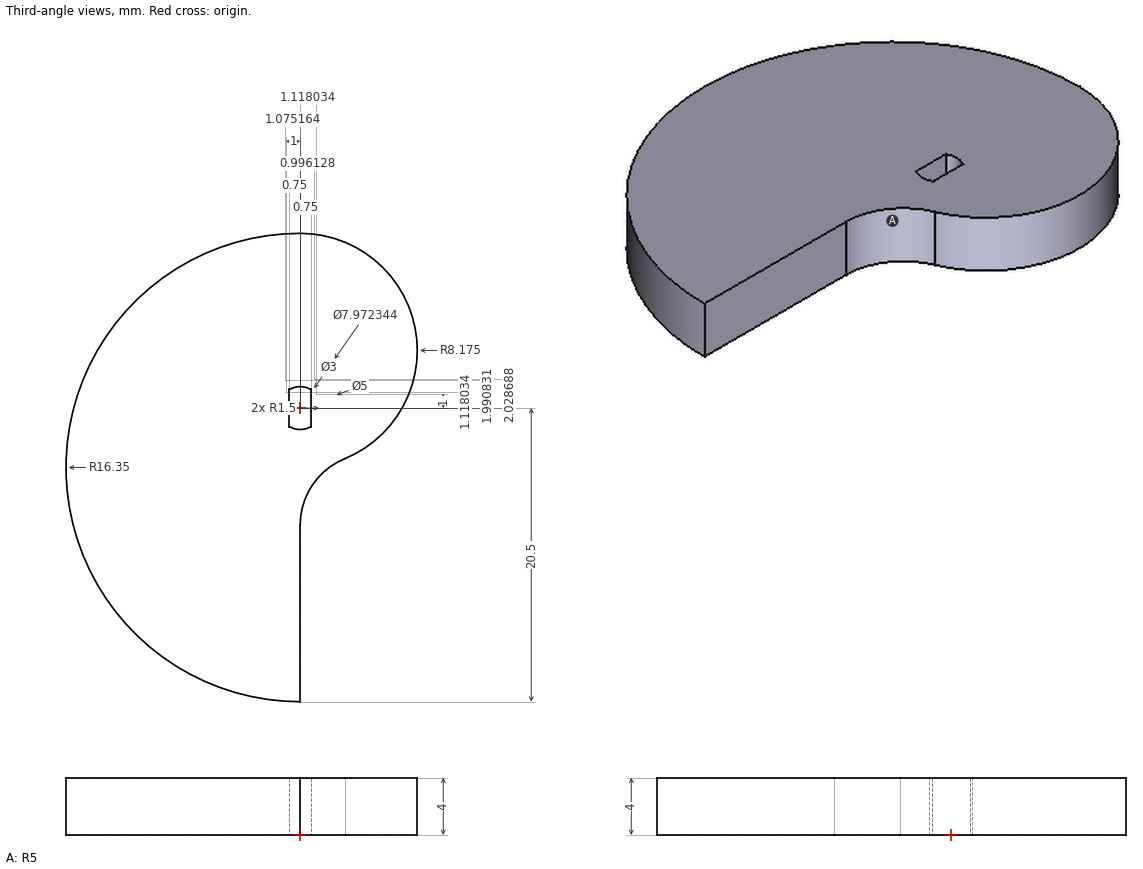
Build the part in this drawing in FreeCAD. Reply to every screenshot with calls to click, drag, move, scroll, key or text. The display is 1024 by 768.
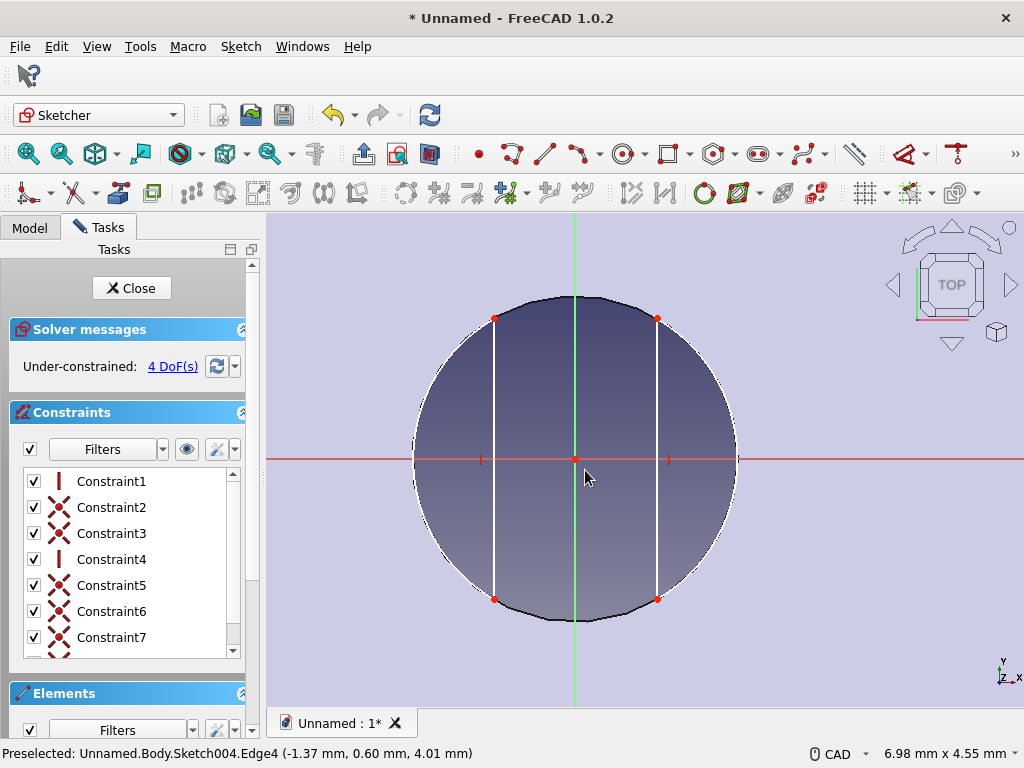
click(724, 525)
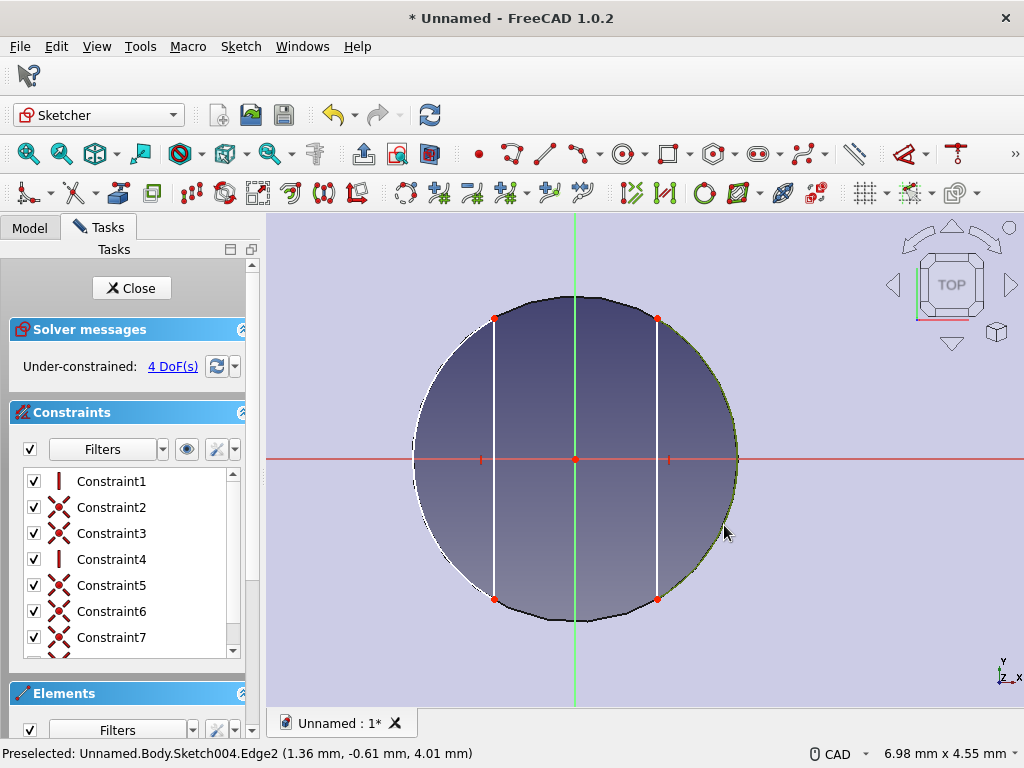
click(427, 393)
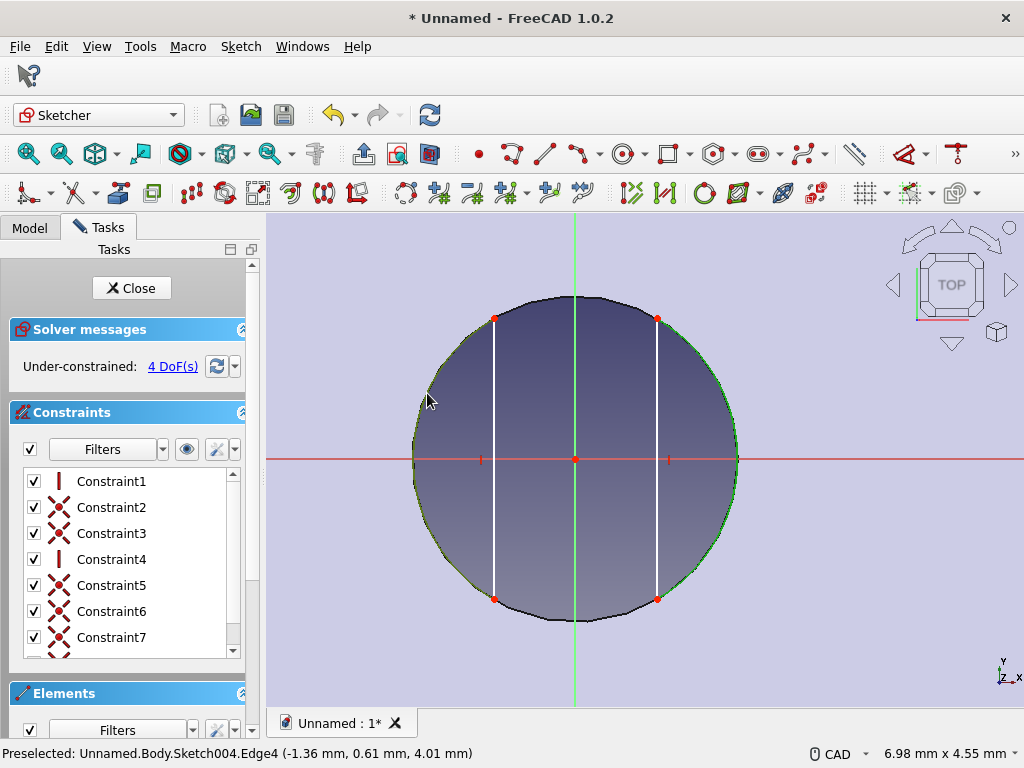
key(e)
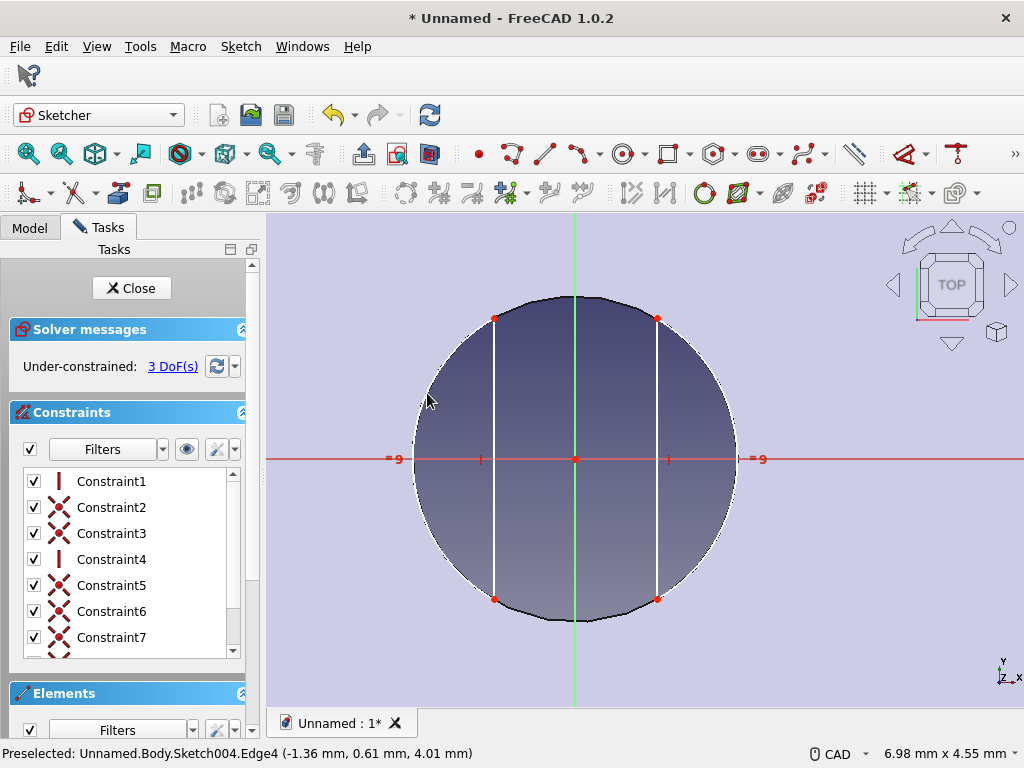
key(d)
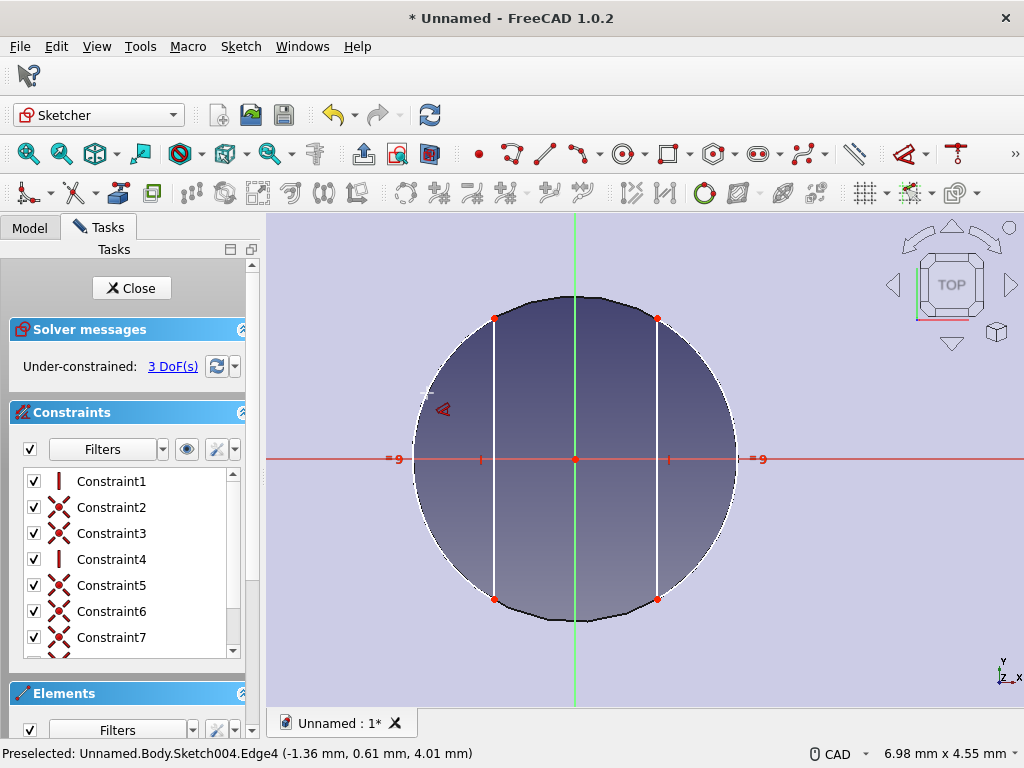
click(724, 525)
click(753, 538)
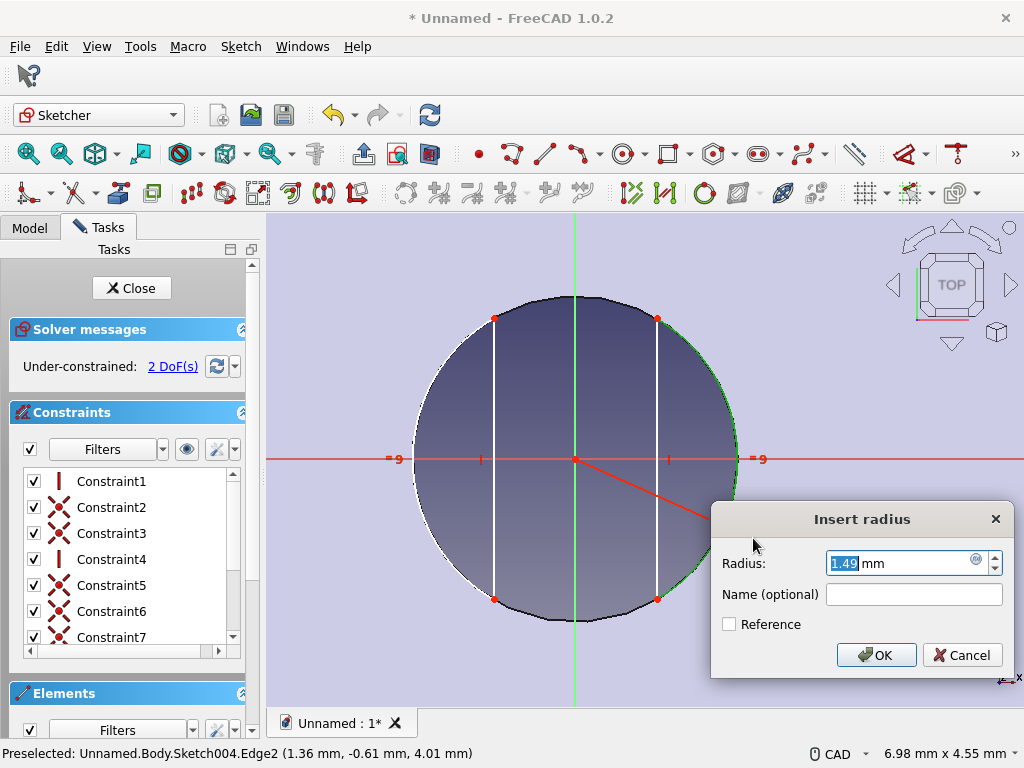
text(1.5)
key(Return)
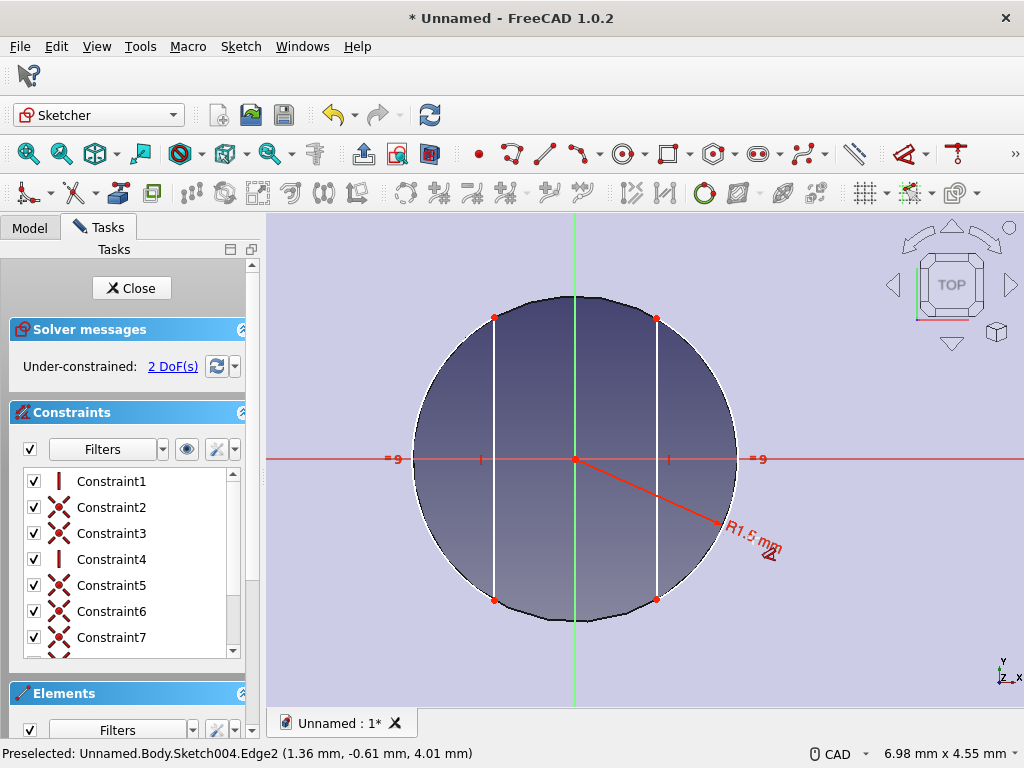
click(657, 318)
click(616, 284)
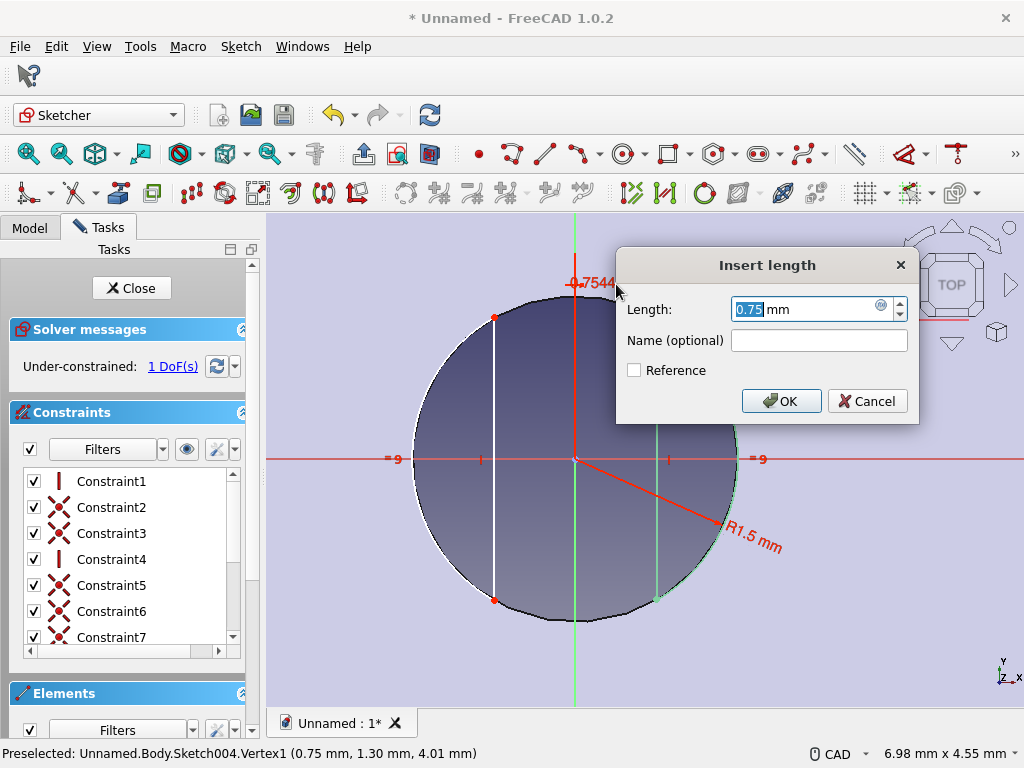
text(0.75)
key(Return)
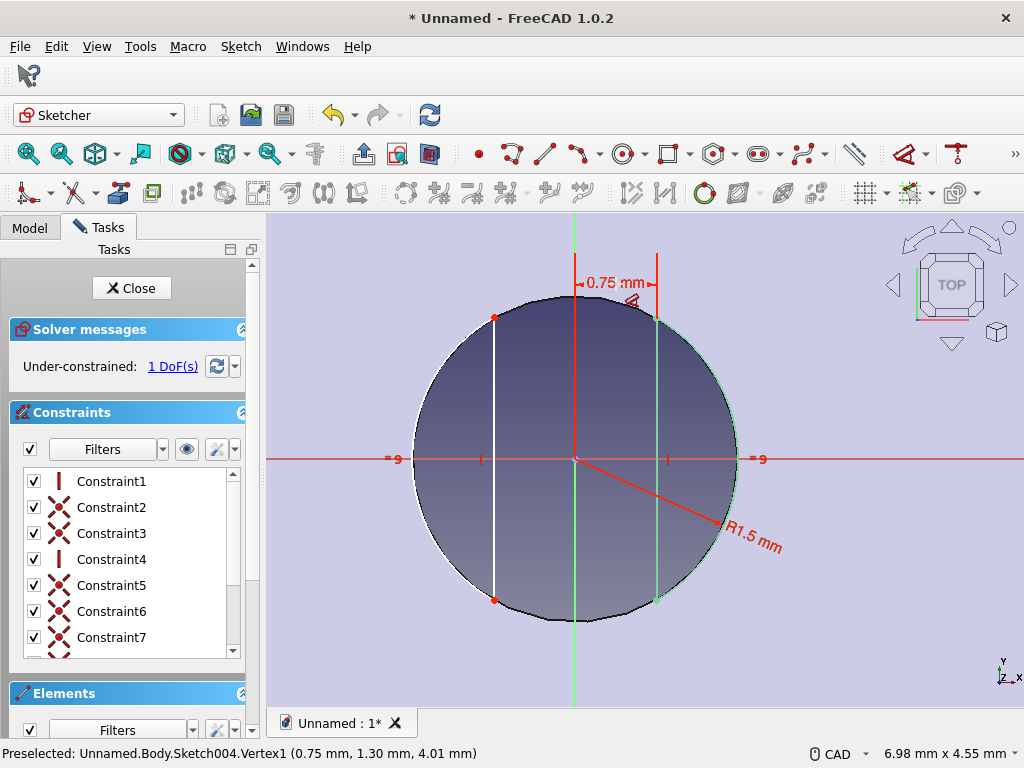
click(494, 600)
click(535, 634)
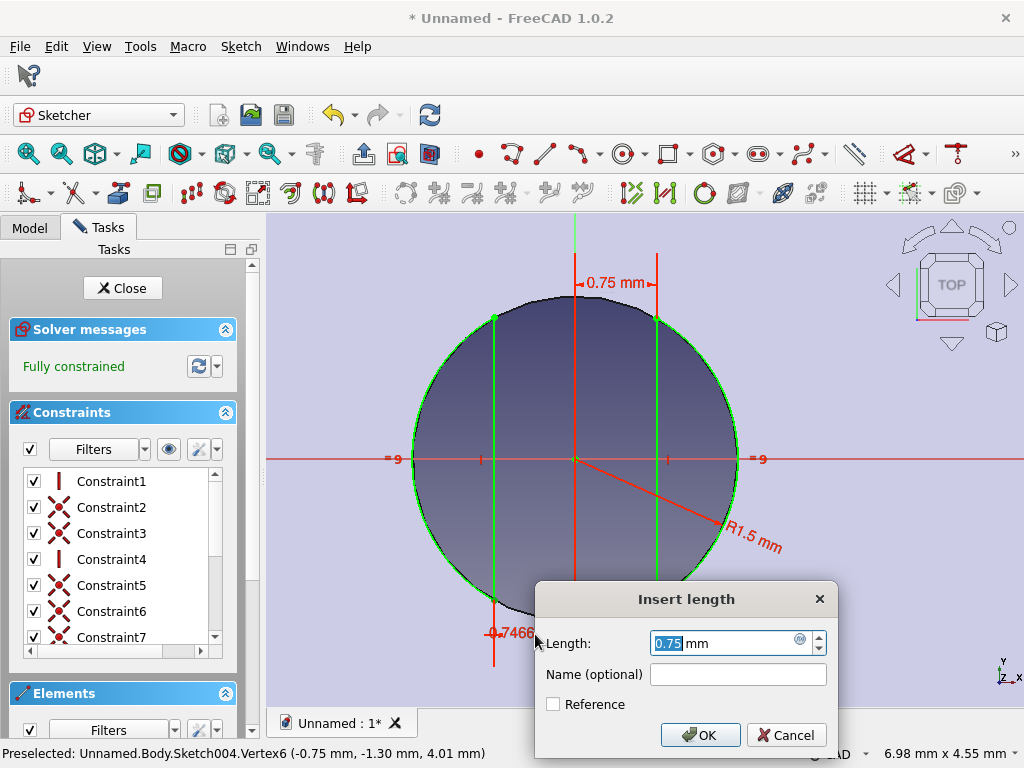
text(0.75)
key(Return)
key(Escape)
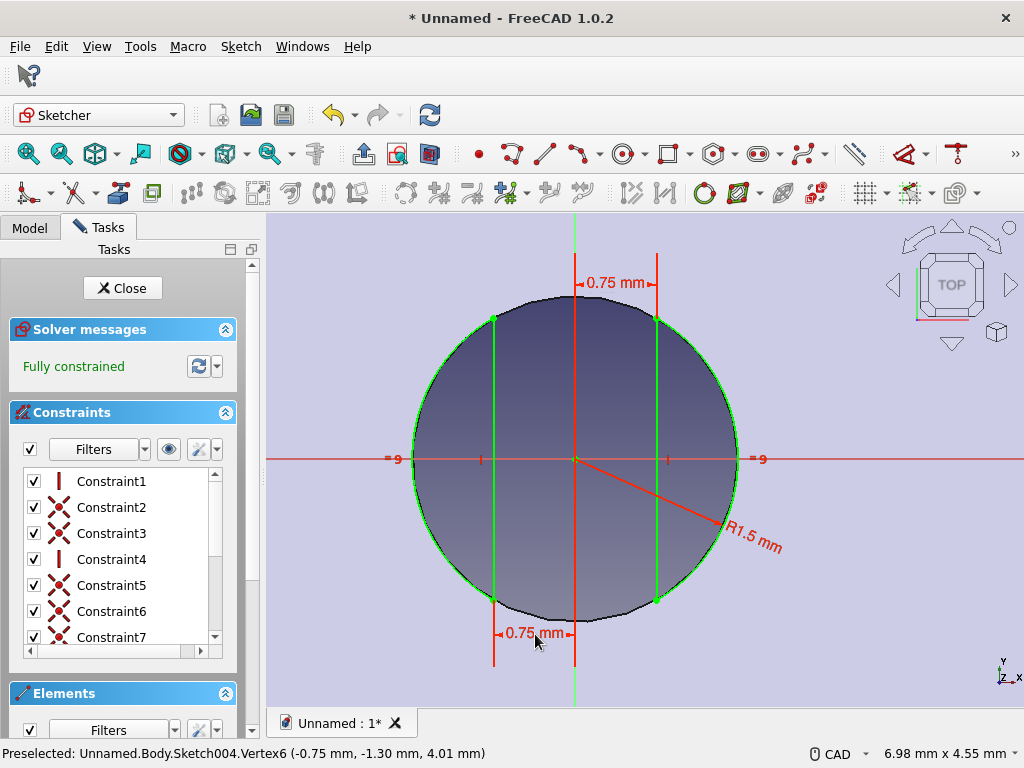
click(123, 288)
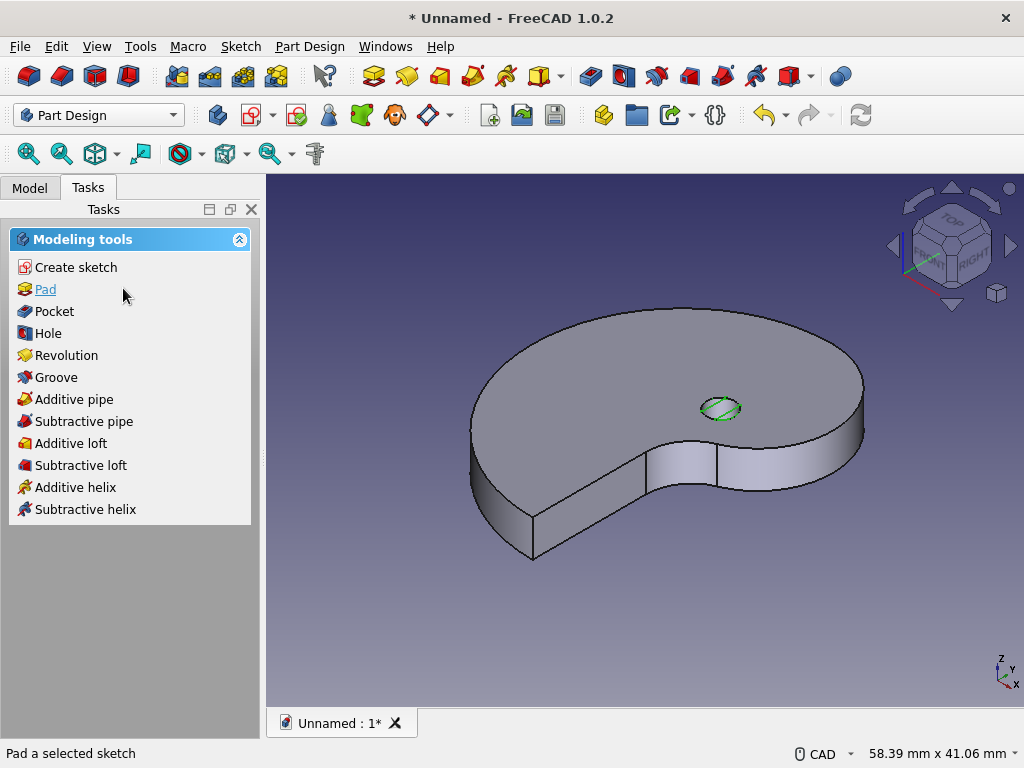
click(374, 76)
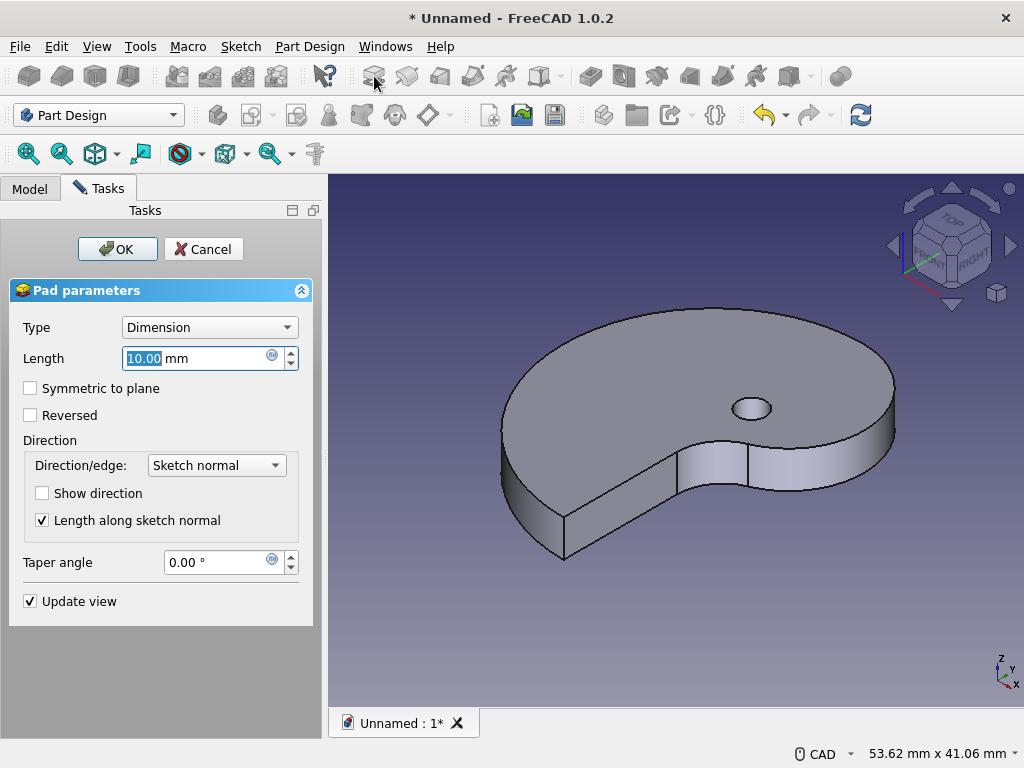
text(4)
key(Tab)